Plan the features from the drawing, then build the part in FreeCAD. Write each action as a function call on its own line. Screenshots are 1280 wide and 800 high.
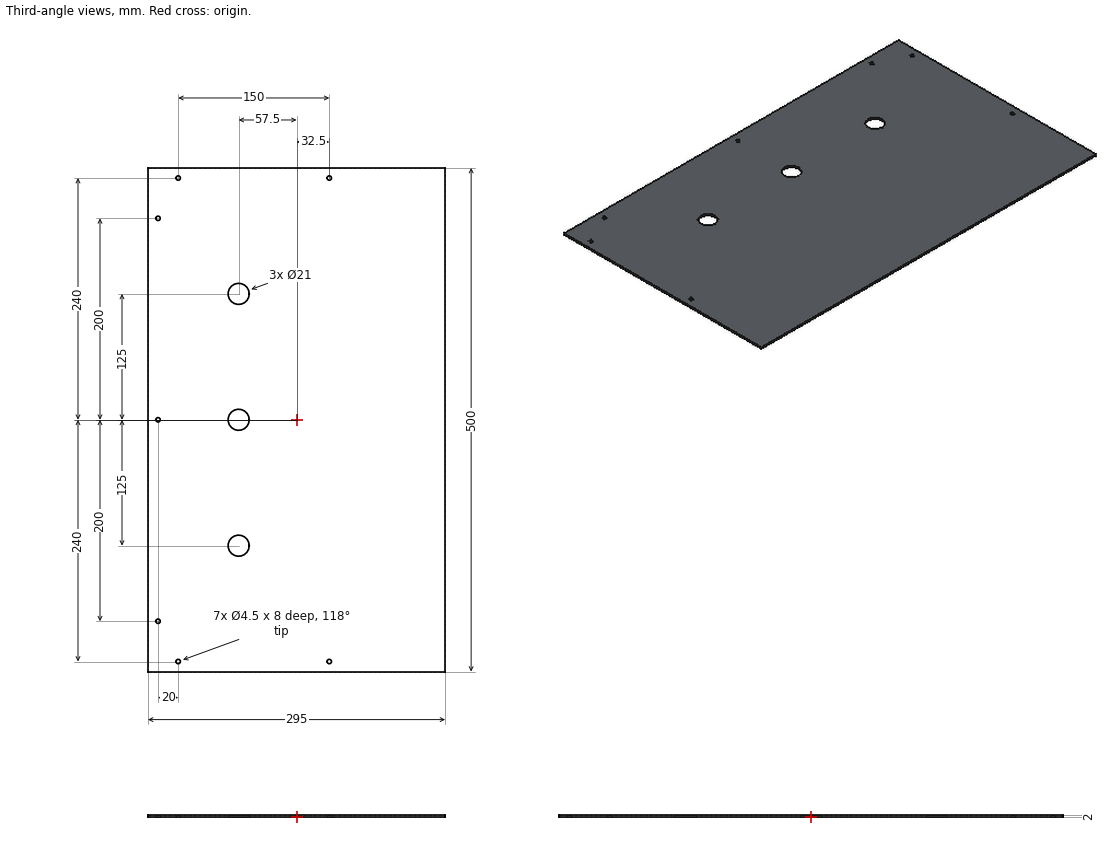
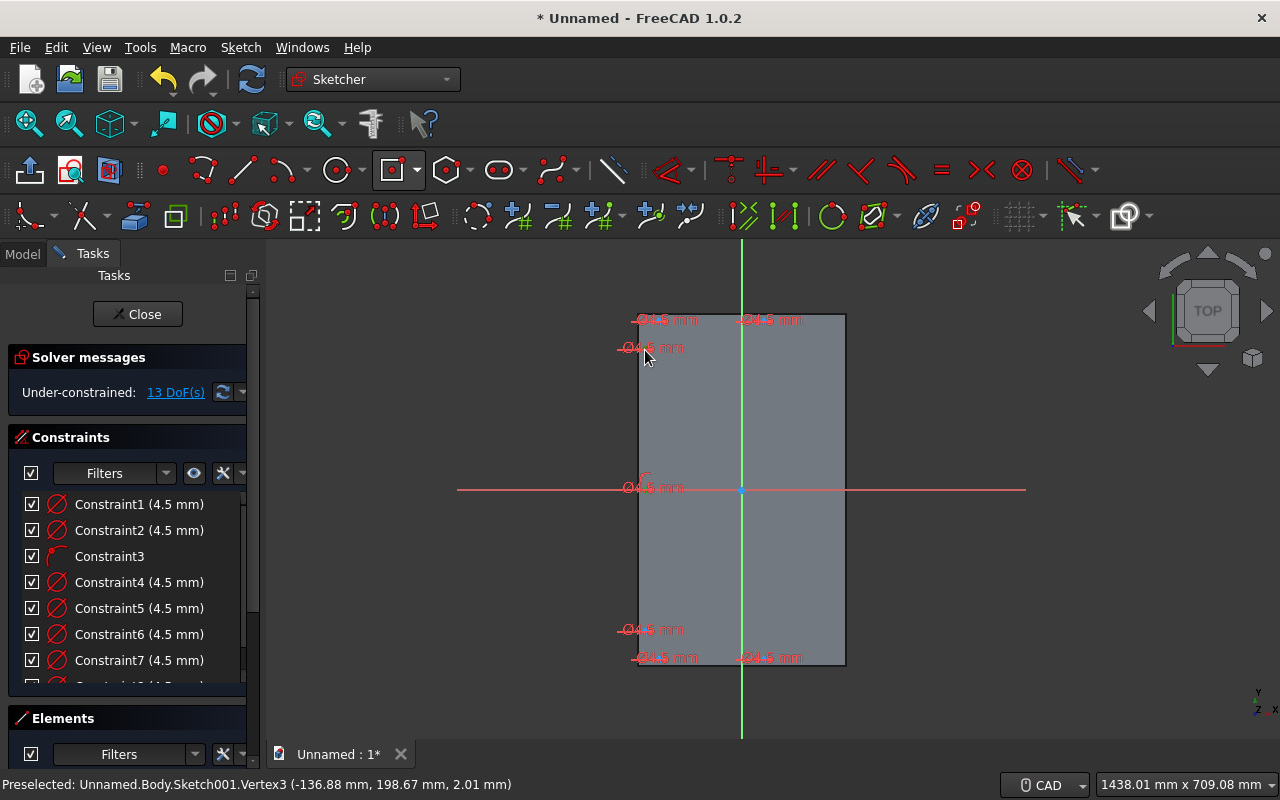
click(796, 170)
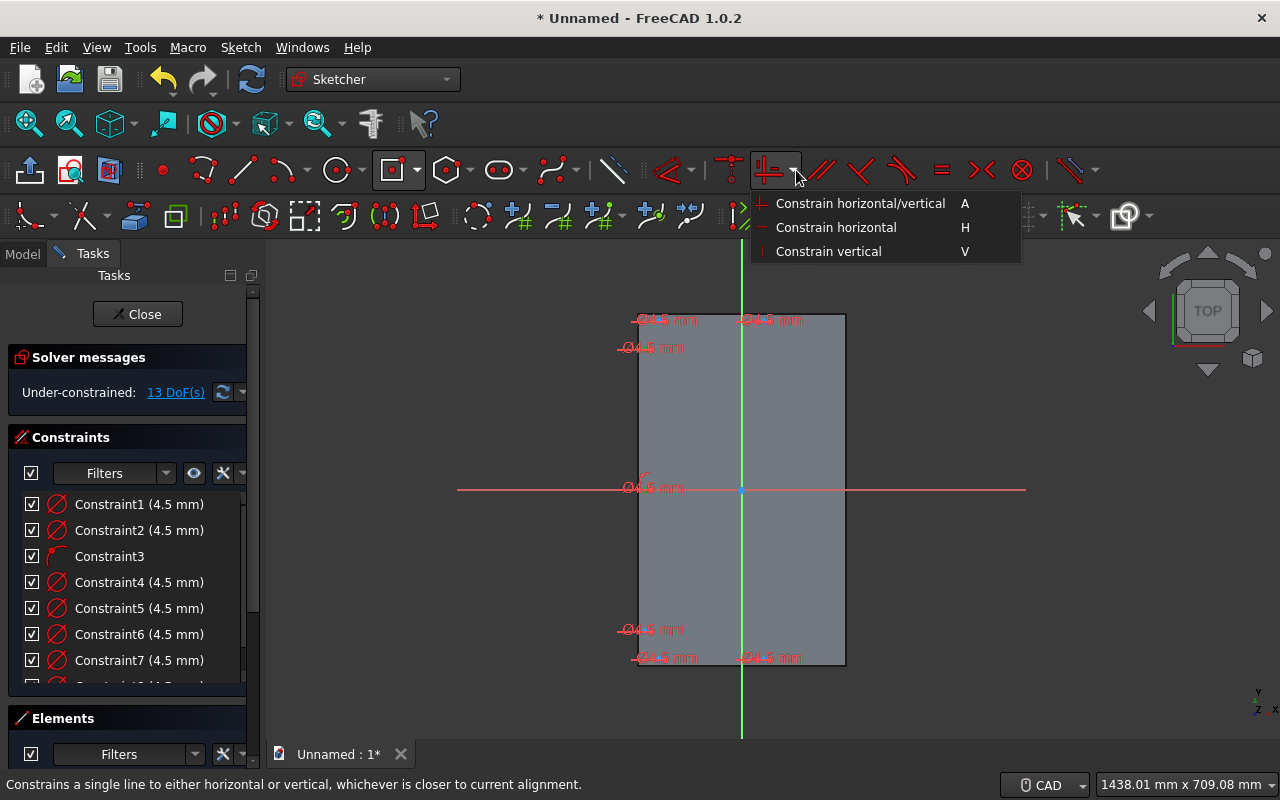
click(886, 251)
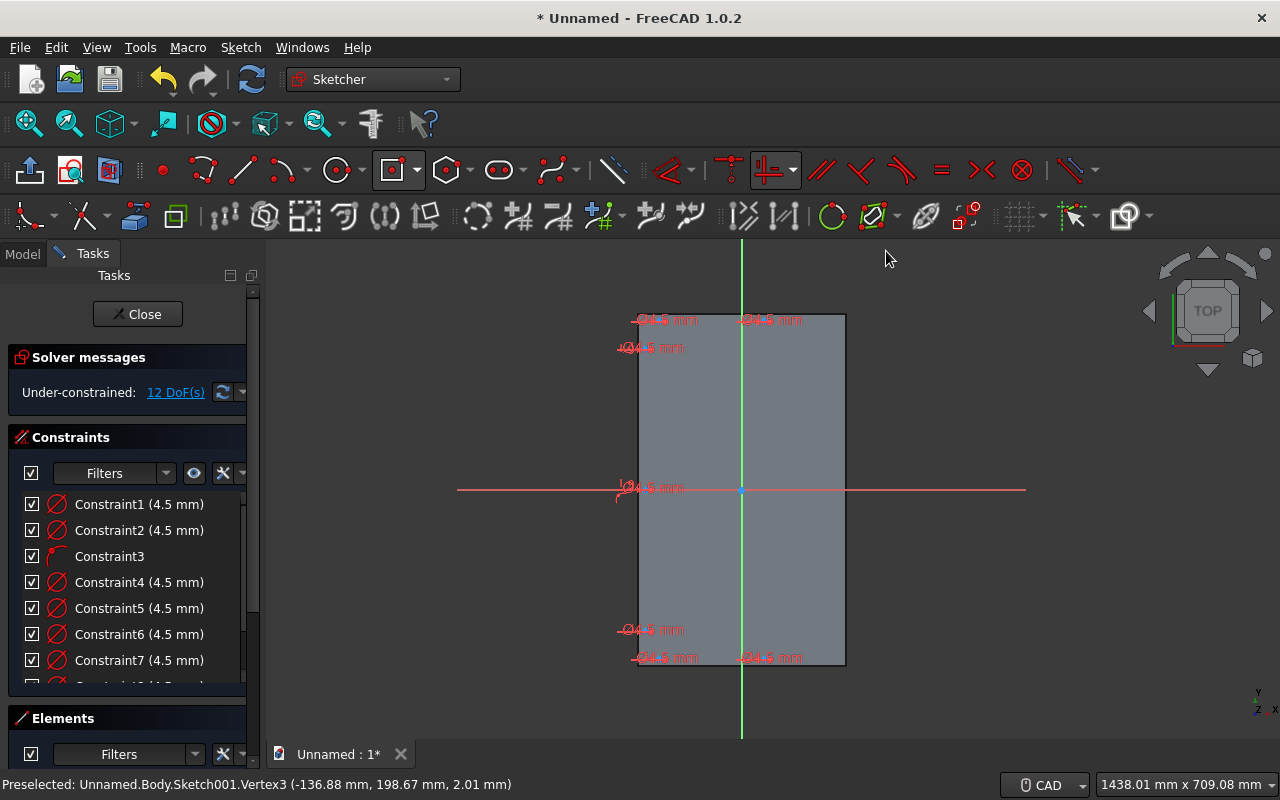
click(645, 490)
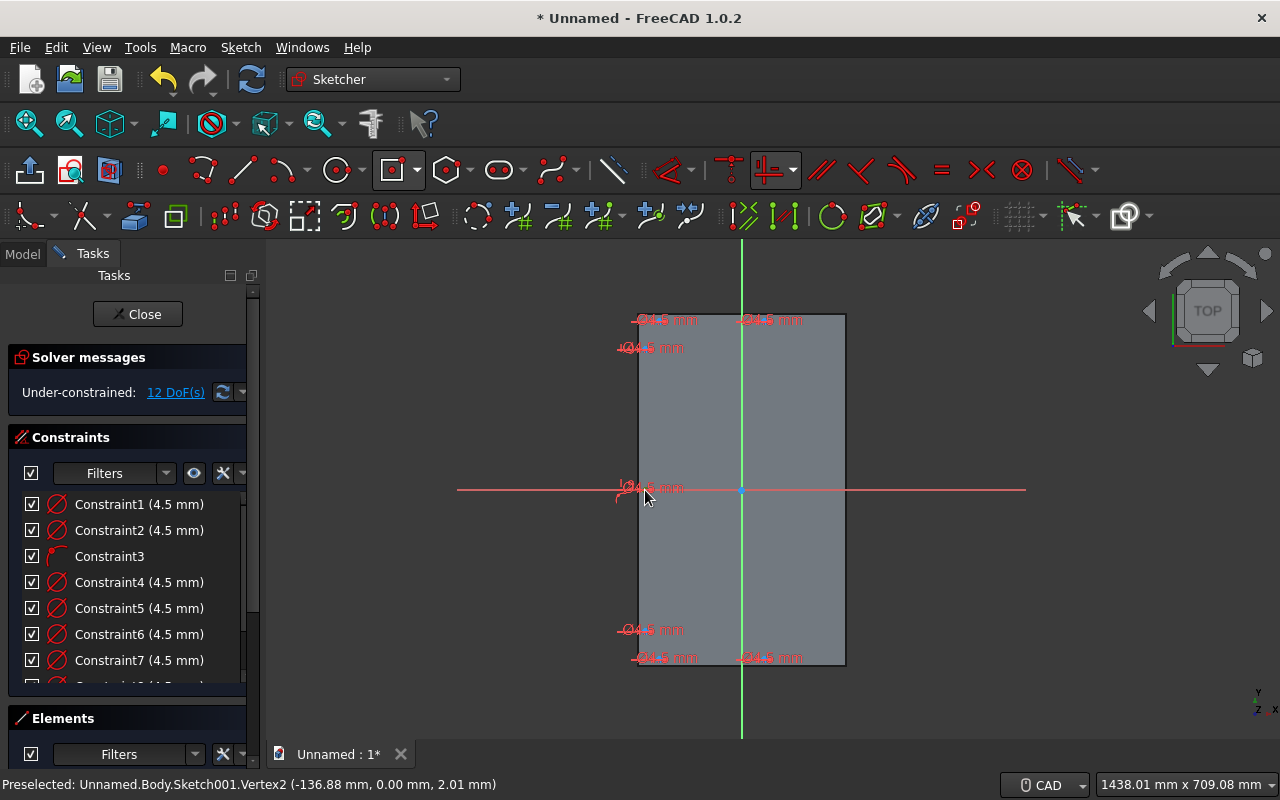
click(645, 632)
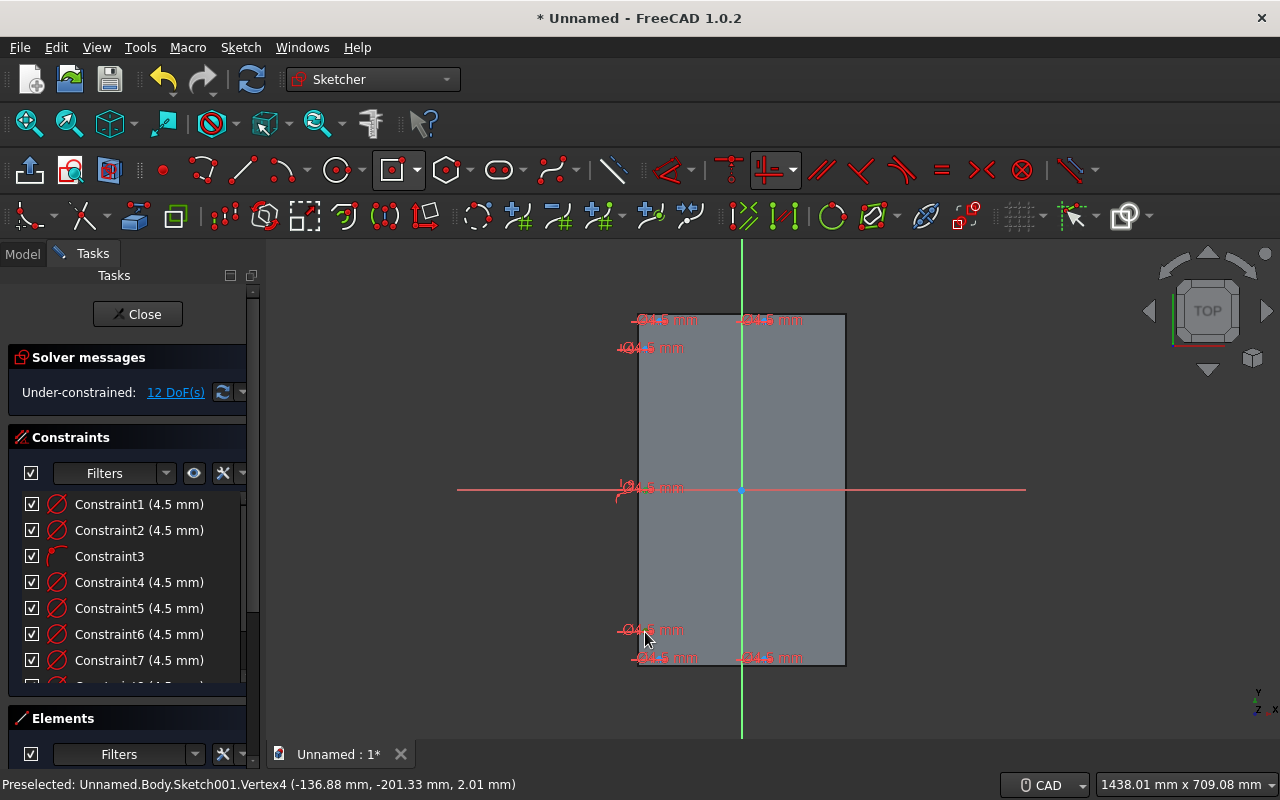
key(v)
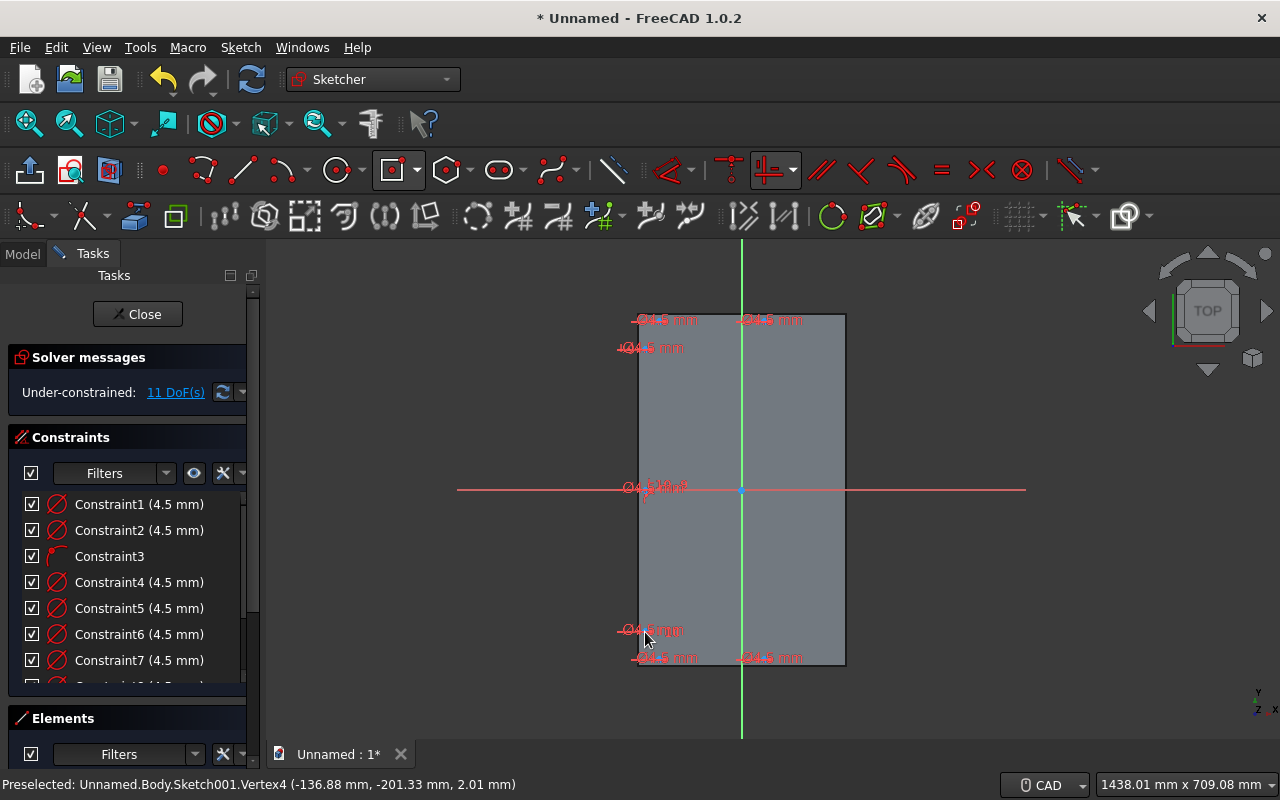
click(659, 660)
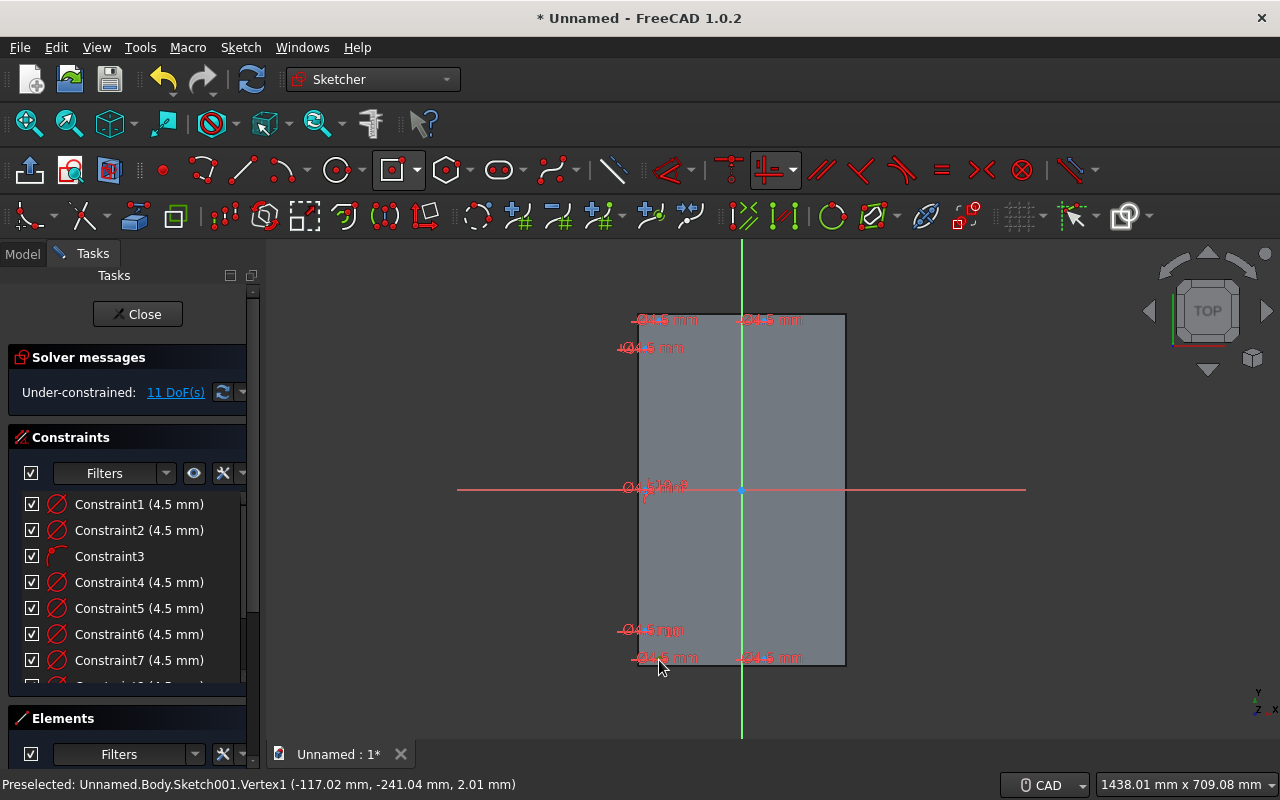
click(659, 322)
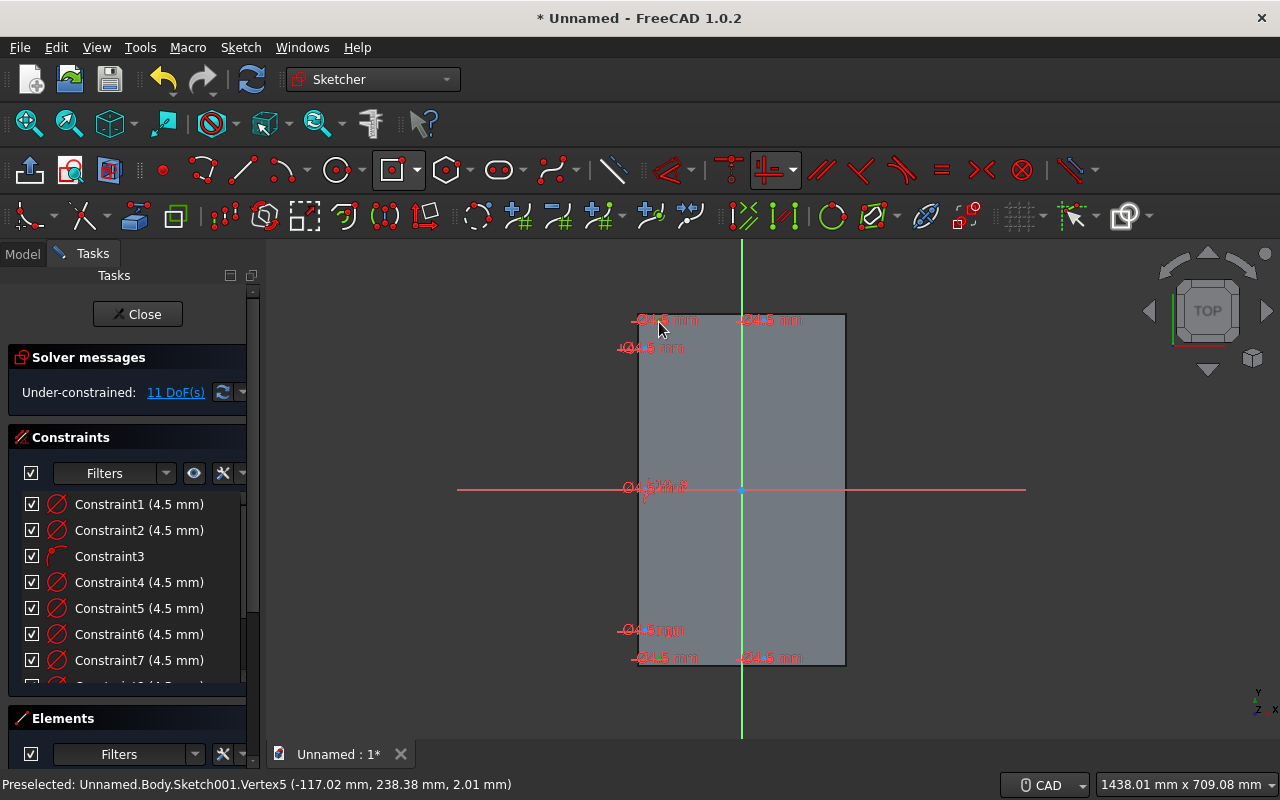
click(796, 170)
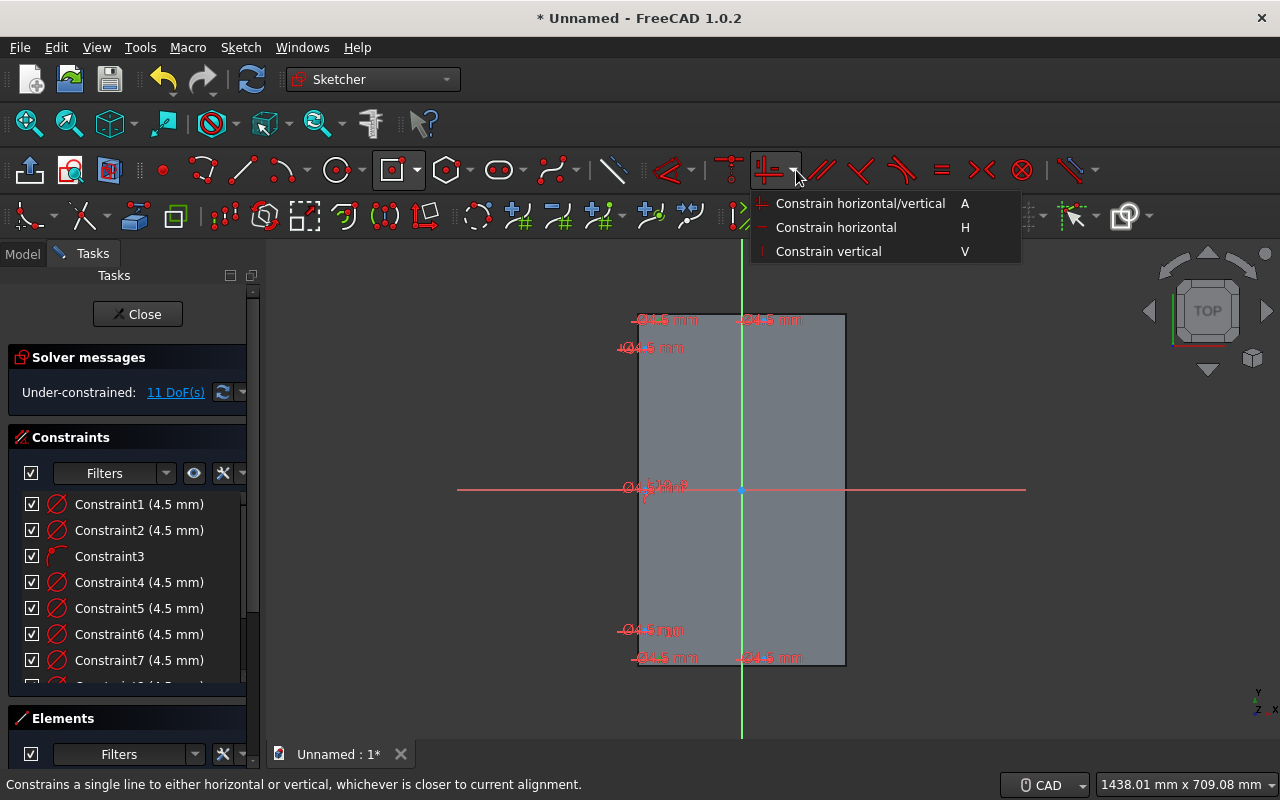
click(886, 251)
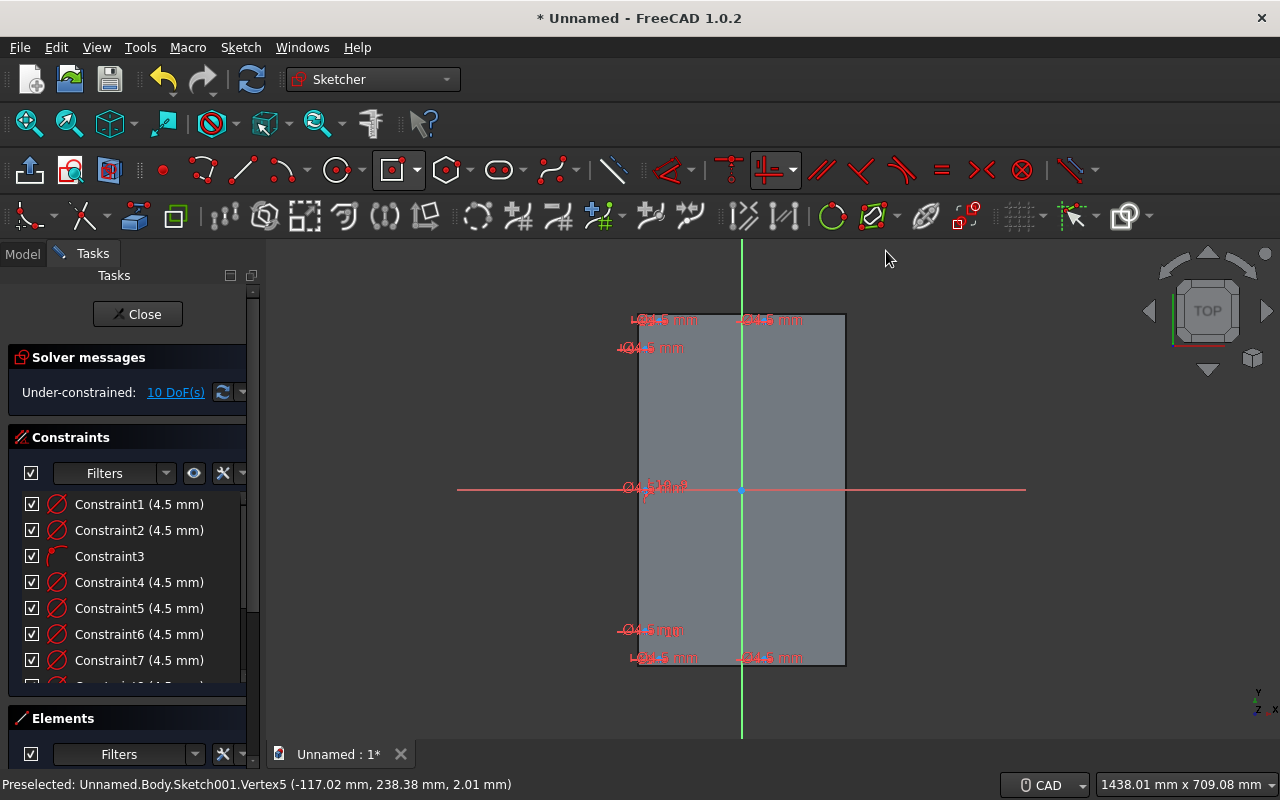
click(659, 322)